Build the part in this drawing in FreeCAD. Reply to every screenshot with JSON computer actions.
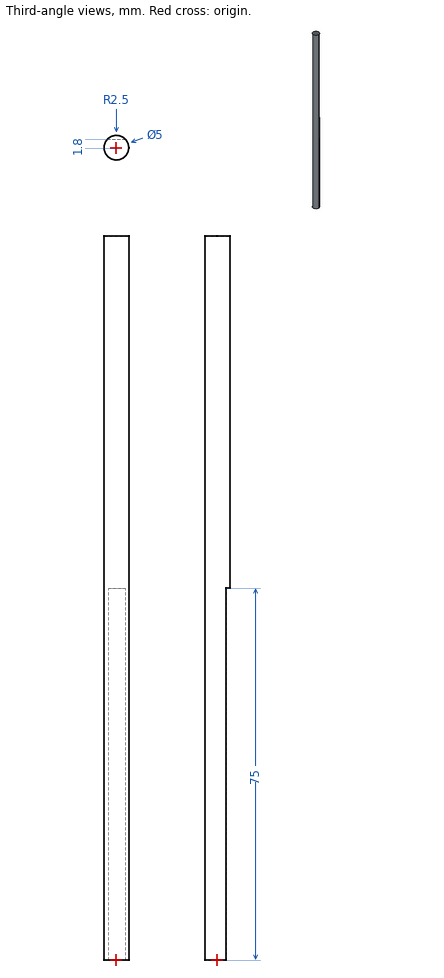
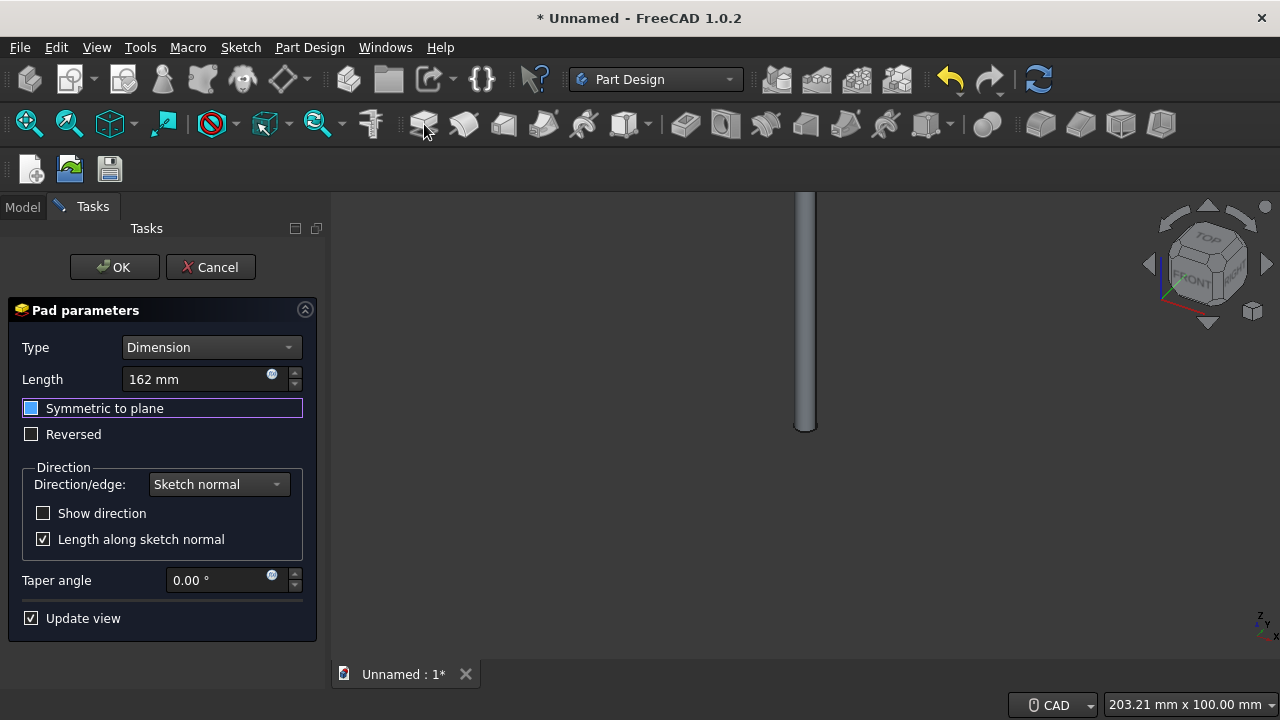
{"action": "left_click", "coordinate": [115, 267]}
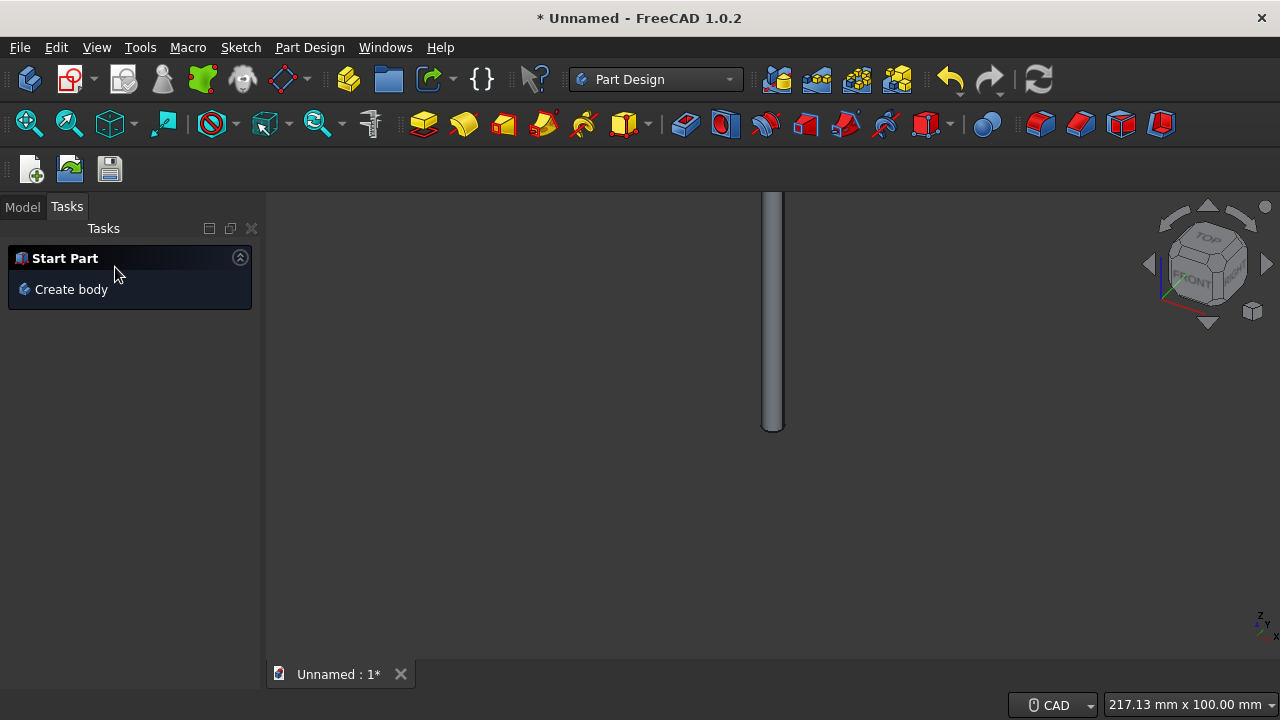
{"action": "left_click", "coordinate": [30, 124]}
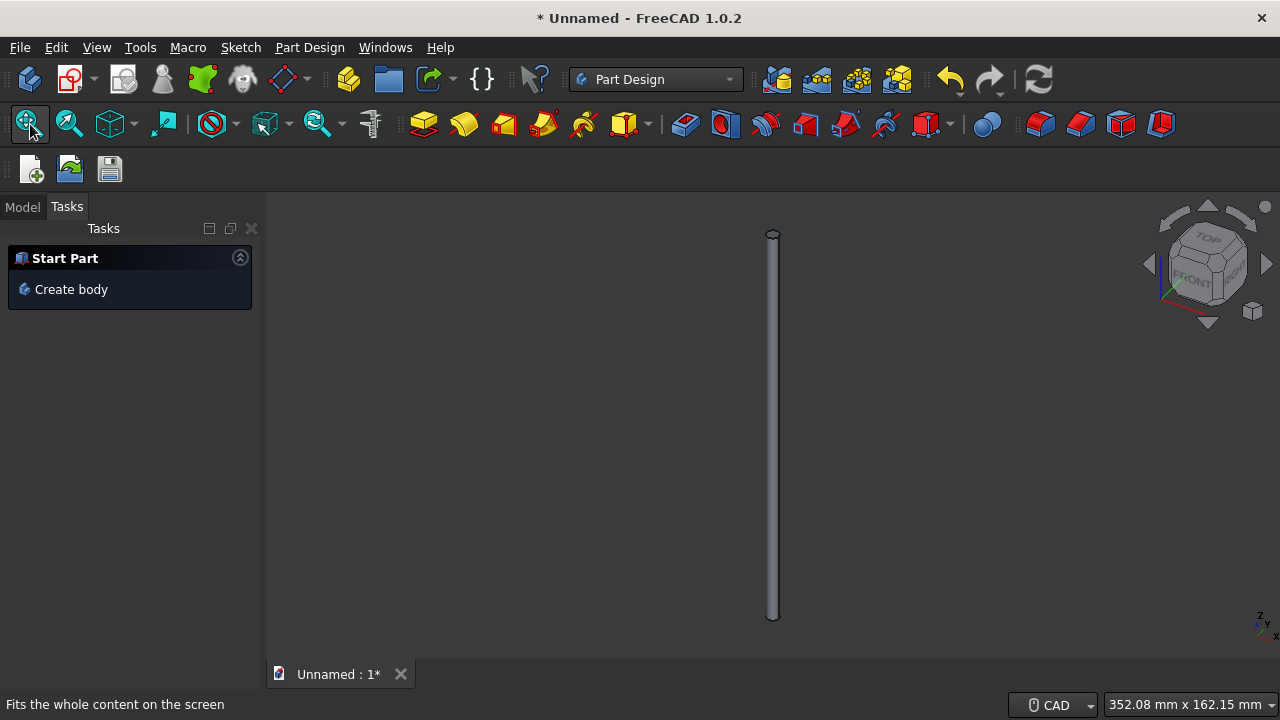
{"action": "left_click", "coordinate": [70, 80]}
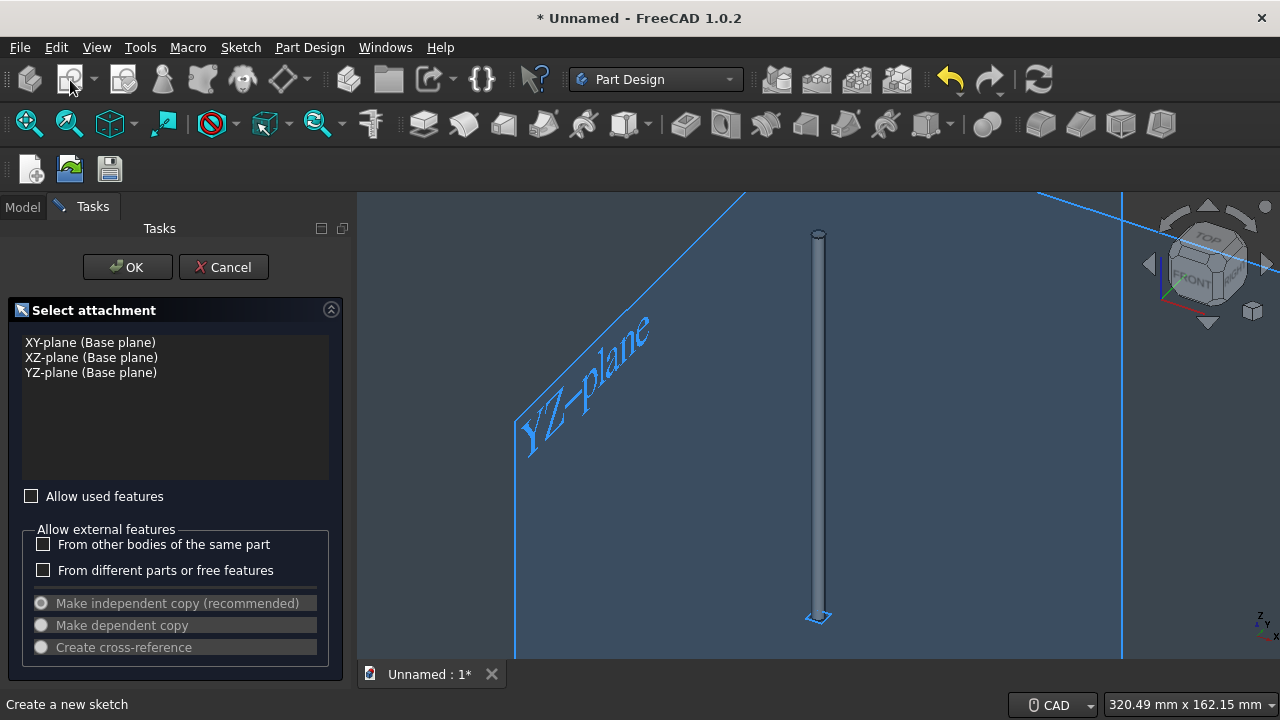
{"action": "left_click", "coordinate": [82, 342]}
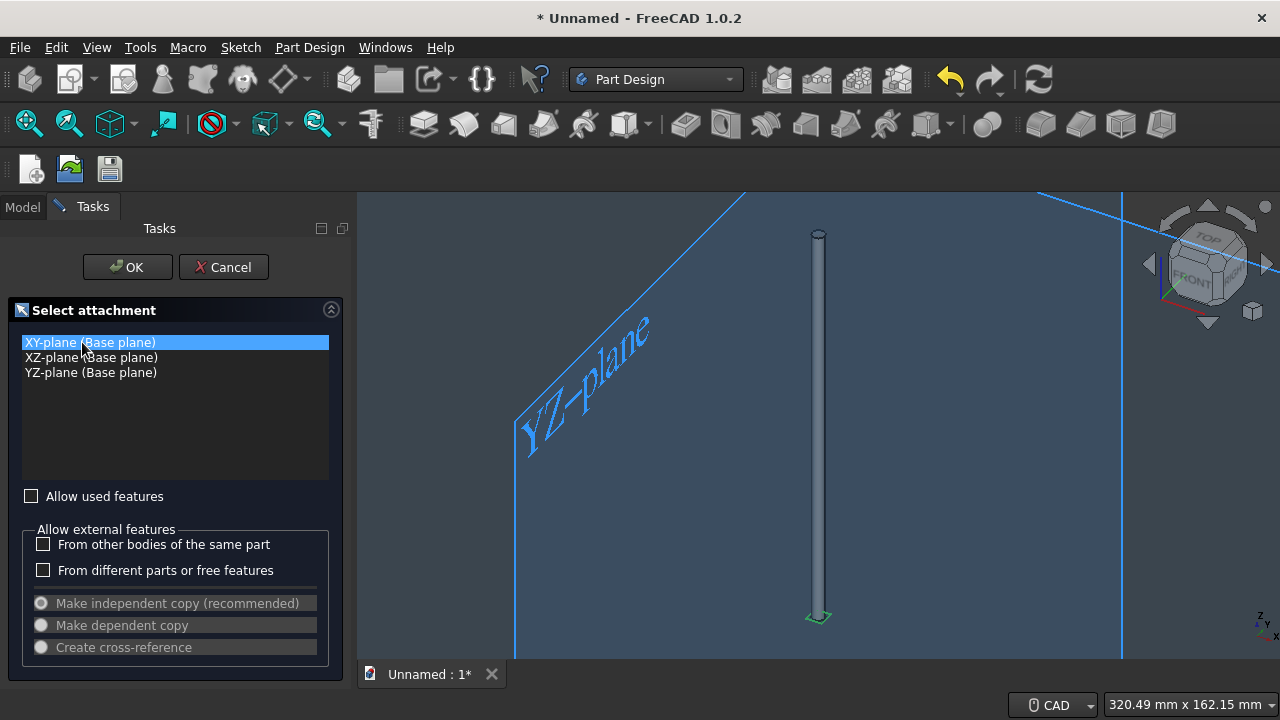
{"action": "left_click", "coordinate": [128, 267]}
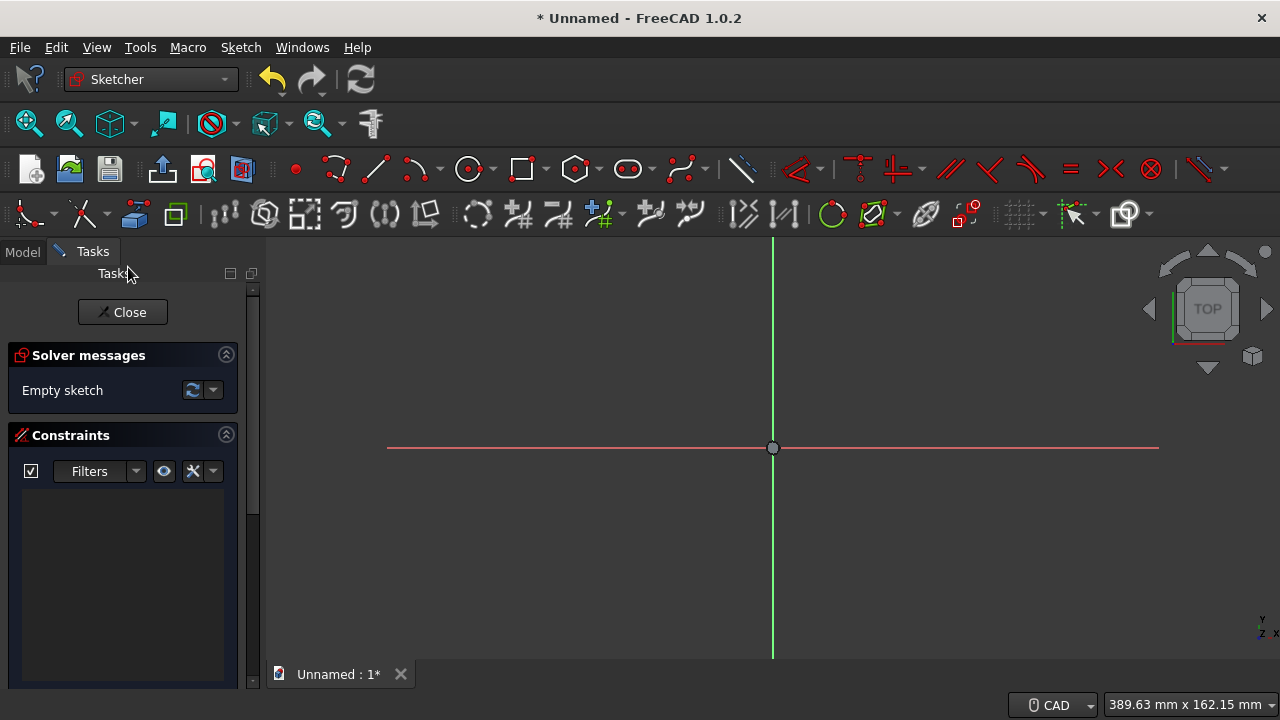
{"action": "key", "text": "q s"}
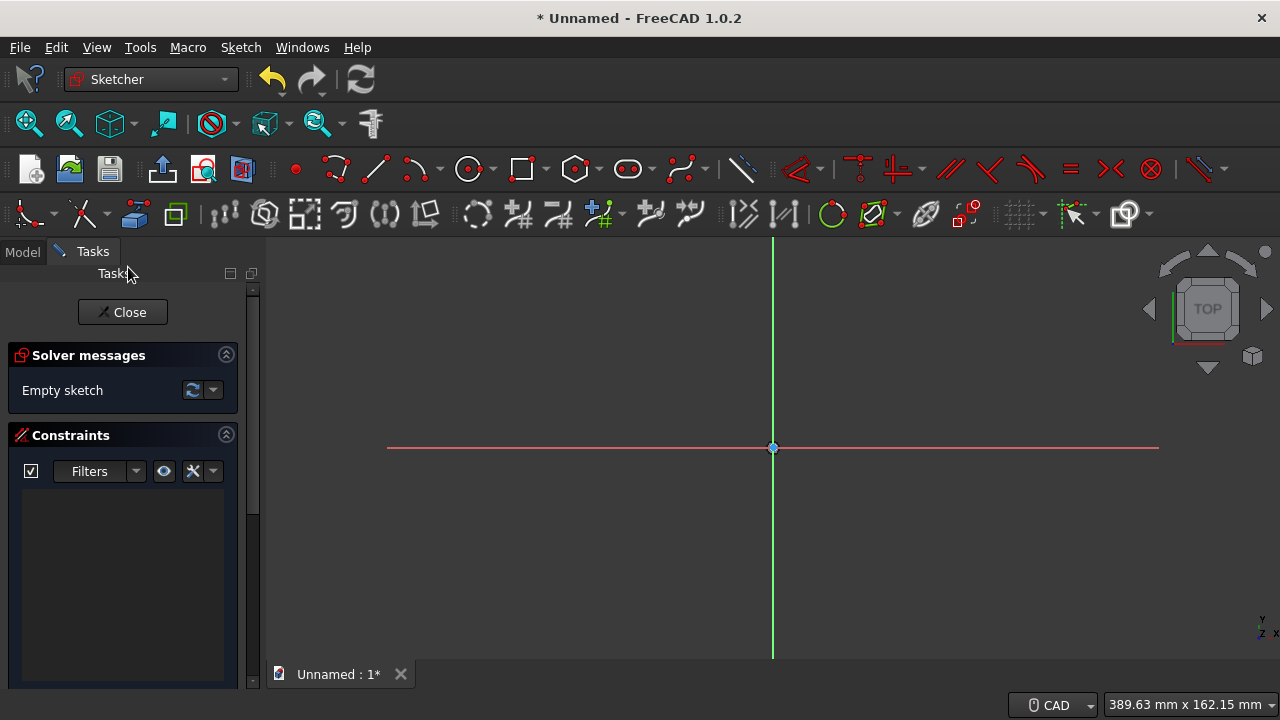
{"action": "scroll", "coordinate": [777, 445], "scroll_direction": "up", "scroll_amount": 15}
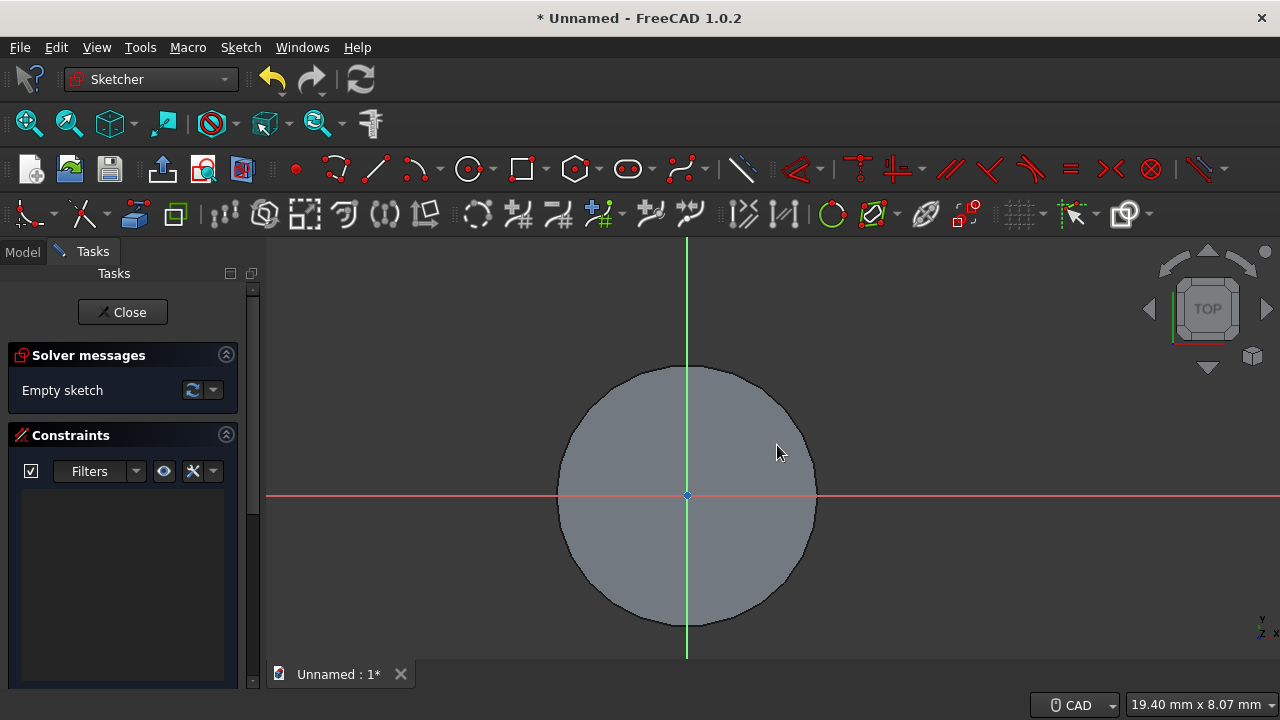
{"action": "scroll", "coordinate": [666, 409], "scroll_direction": "up", "scroll_amount": 3}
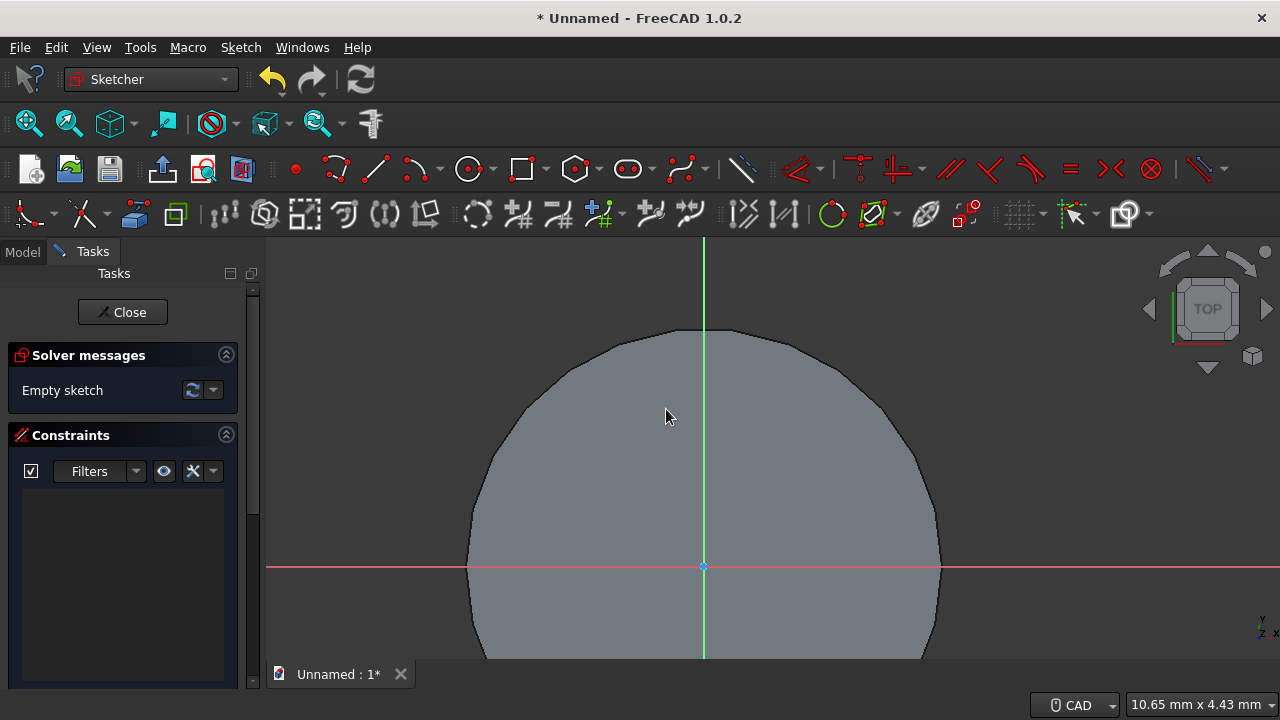
{"action": "left_click", "coordinate": [376, 170]}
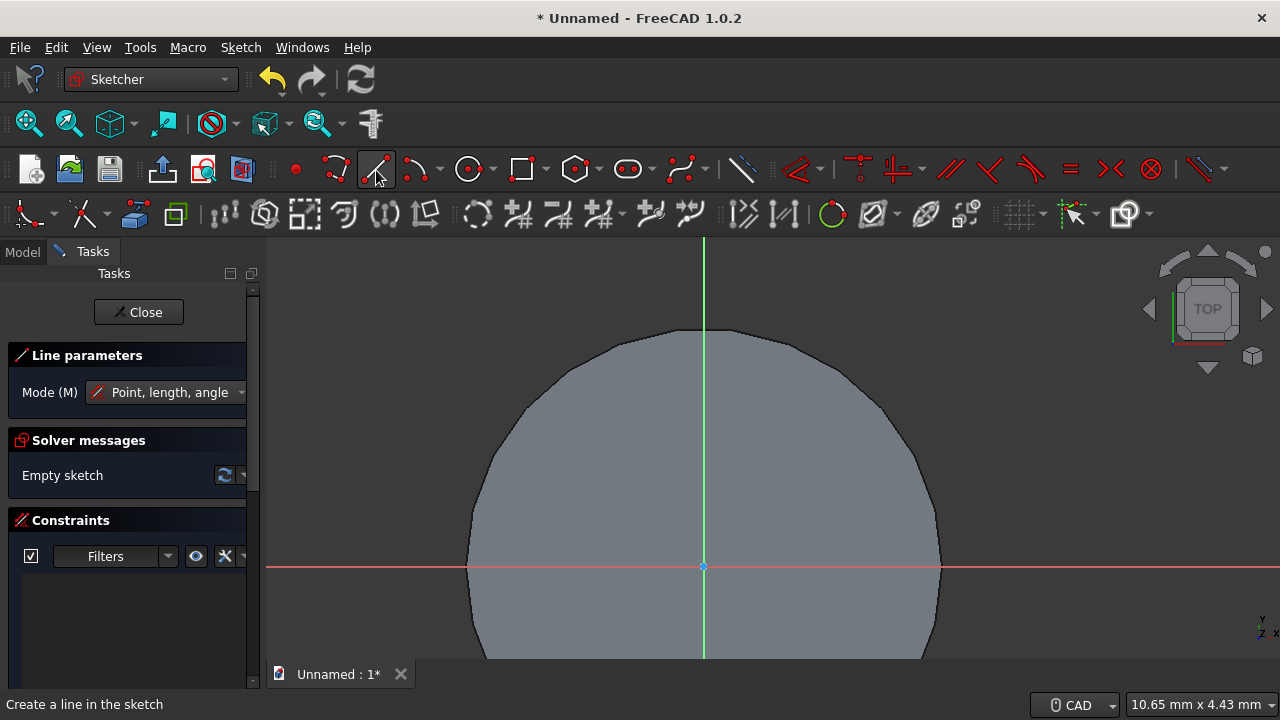
{"action": "left_click", "coordinate": [539, 395]}
{"action": "left_click", "coordinate": [869, 395]}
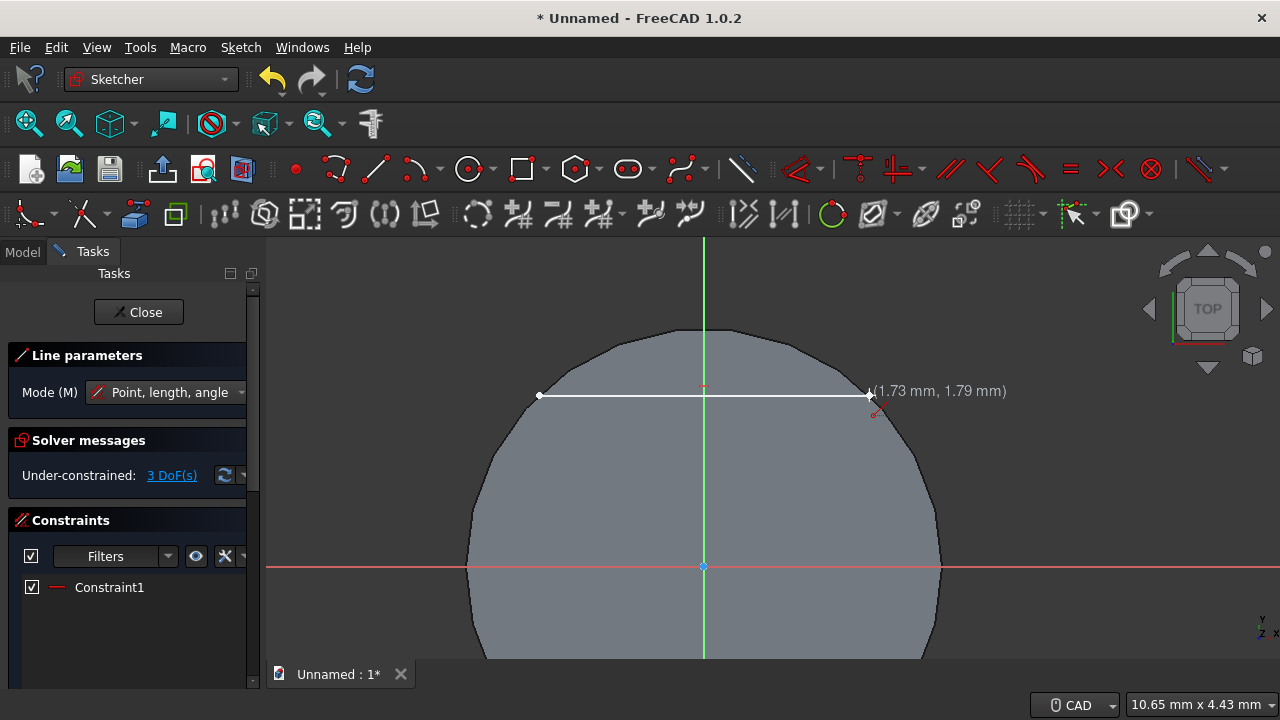
{"action": "key", "text": "g 3 a"}